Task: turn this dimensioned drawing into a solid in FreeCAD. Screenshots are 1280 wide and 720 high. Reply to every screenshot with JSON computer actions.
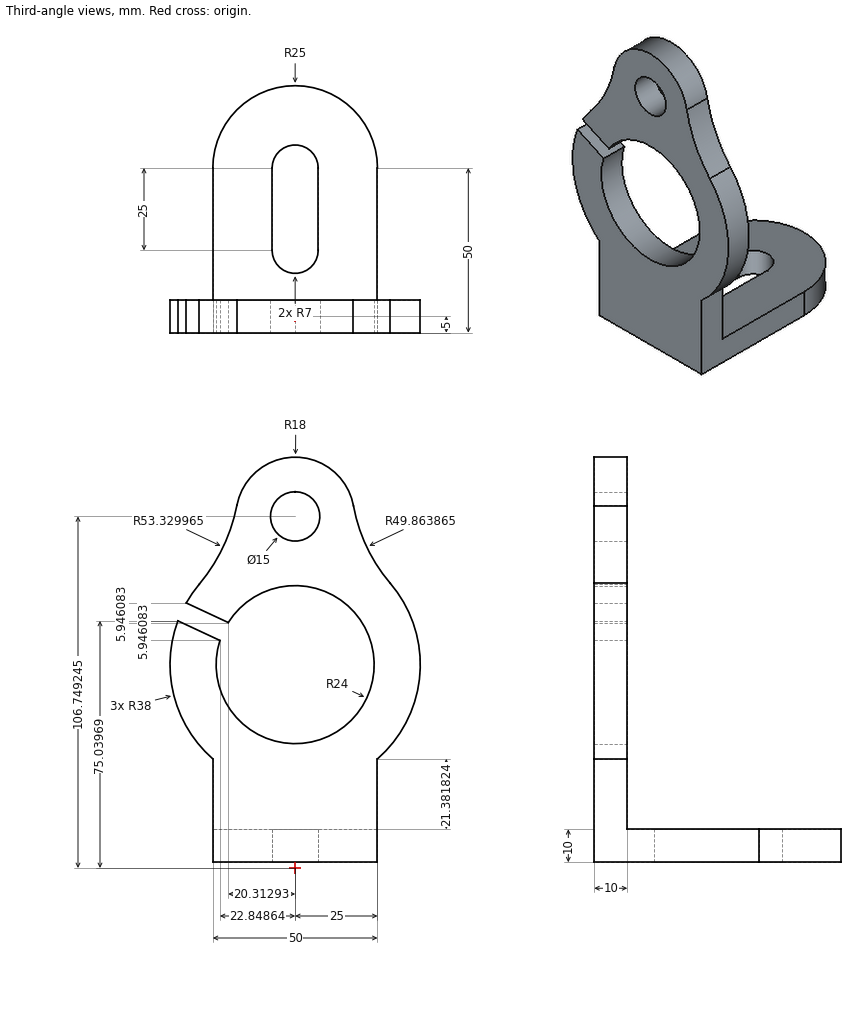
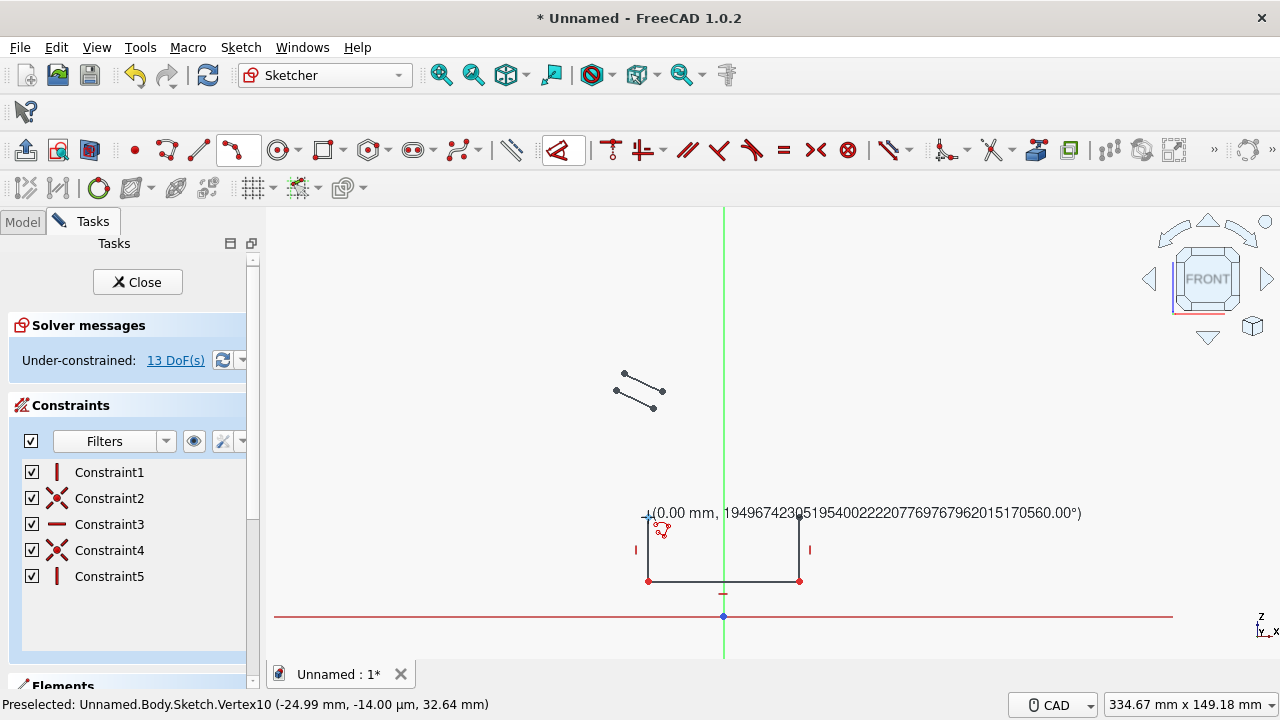
{"action": "left_click", "coordinate": [232, 150]}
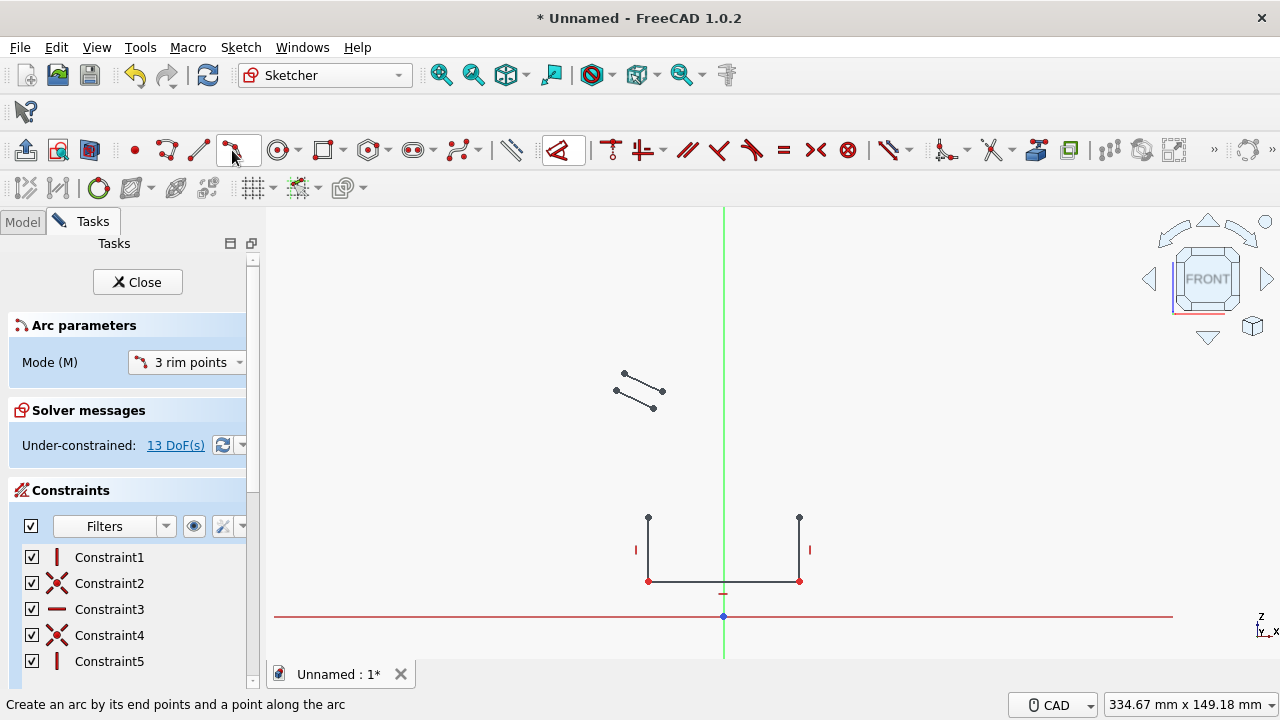
{"action": "left_click", "coordinate": [654, 409]}
{"action": "left_click", "coordinate": [662, 392]}
{"action": "left_click", "coordinate": [790, 461]}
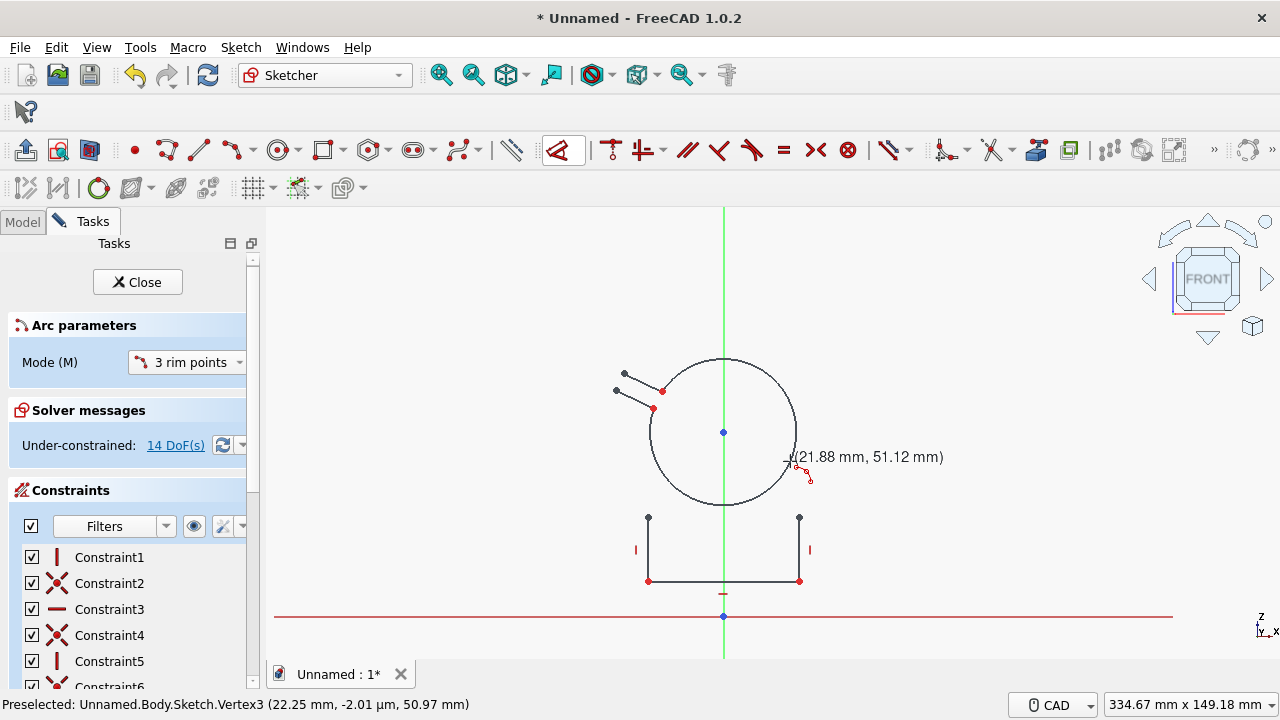
{"action": "left_click", "coordinate": [624, 374]}
{"action": "left_click", "coordinate": [635, 356]}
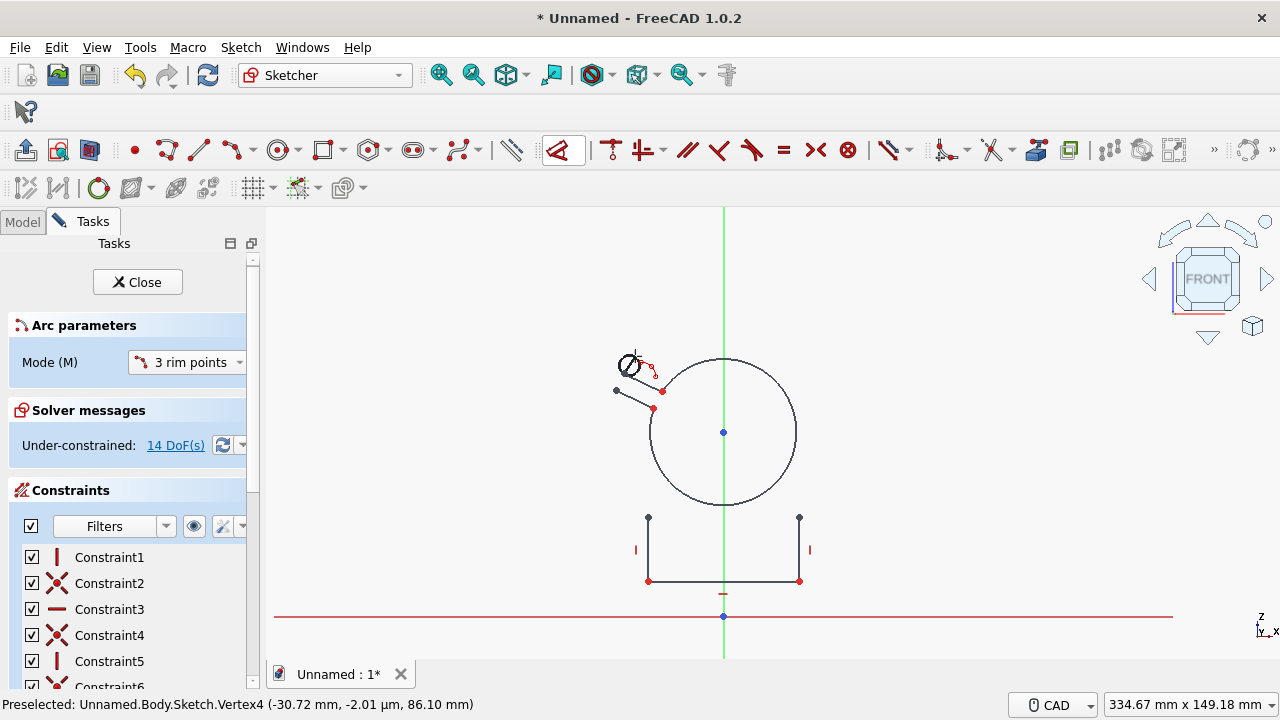
{"action": "scroll", "coordinate": [629, 364], "scroll_direction": "up", "scroll_amount": 18}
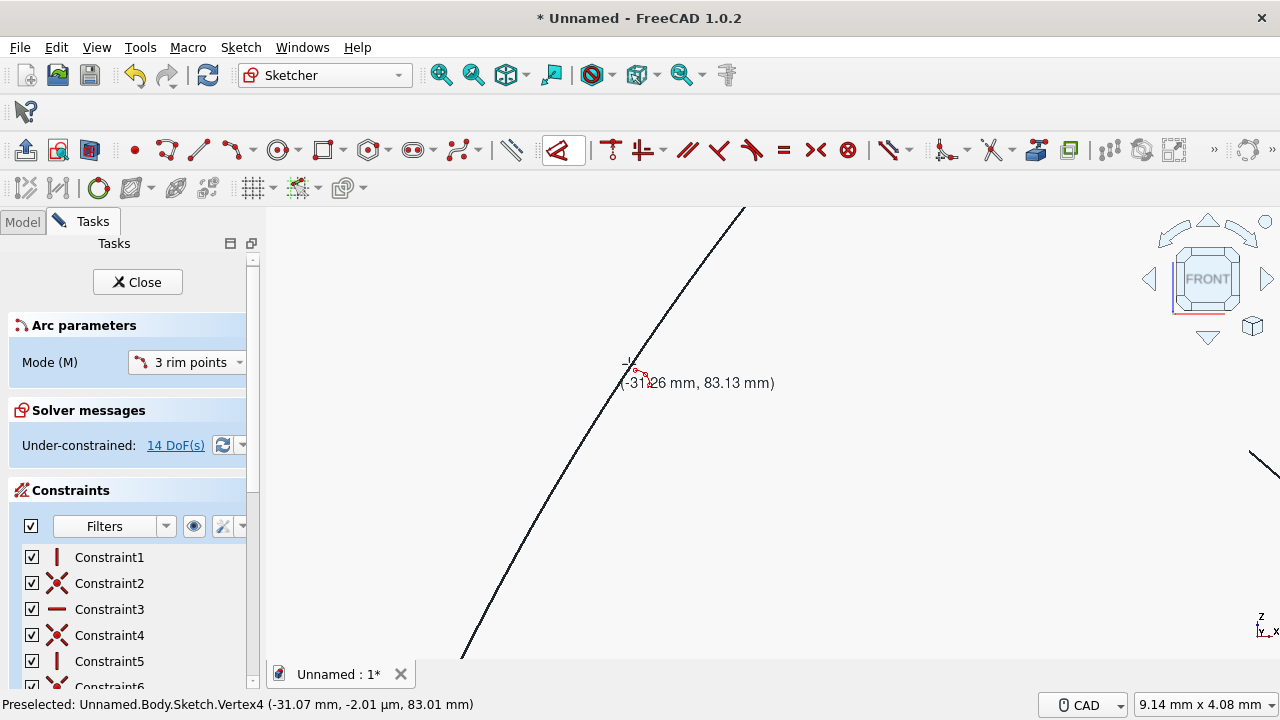
{"action": "left_click", "coordinate": [620, 358]}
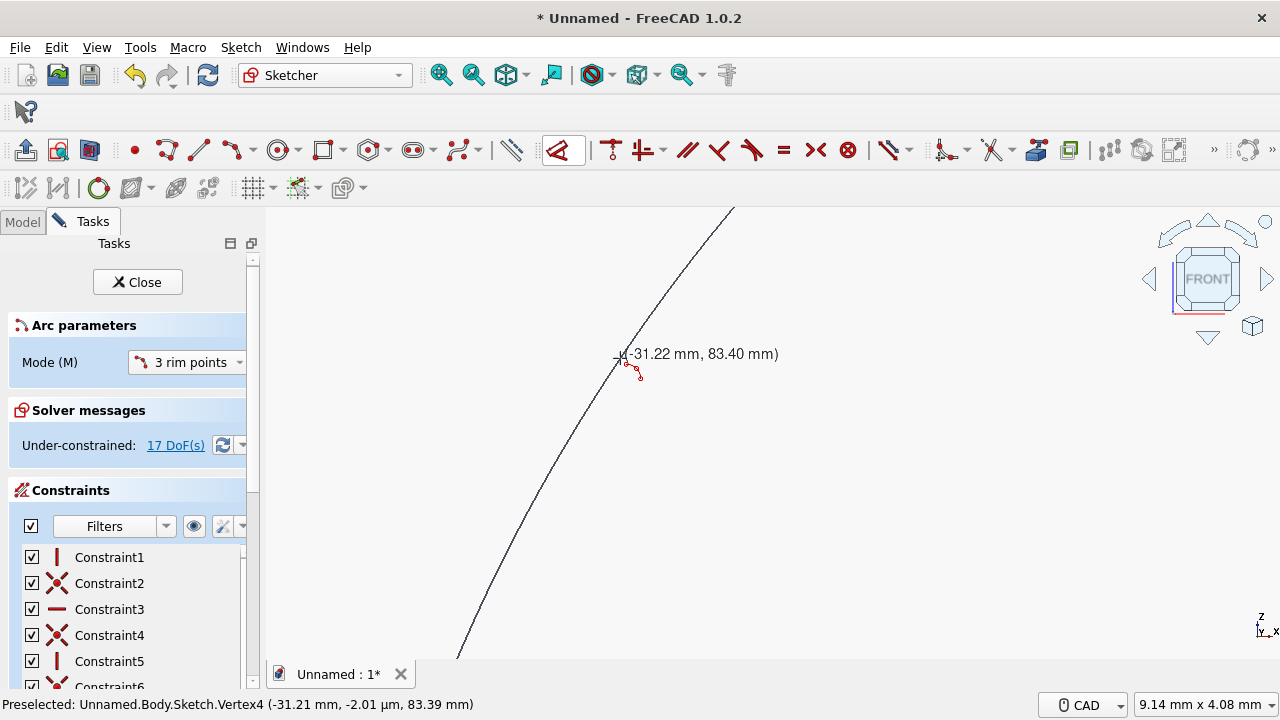
{"action": "scroll", "coordinate": [704, 433], "scroll_direction": "down", "scroll_amount": 15}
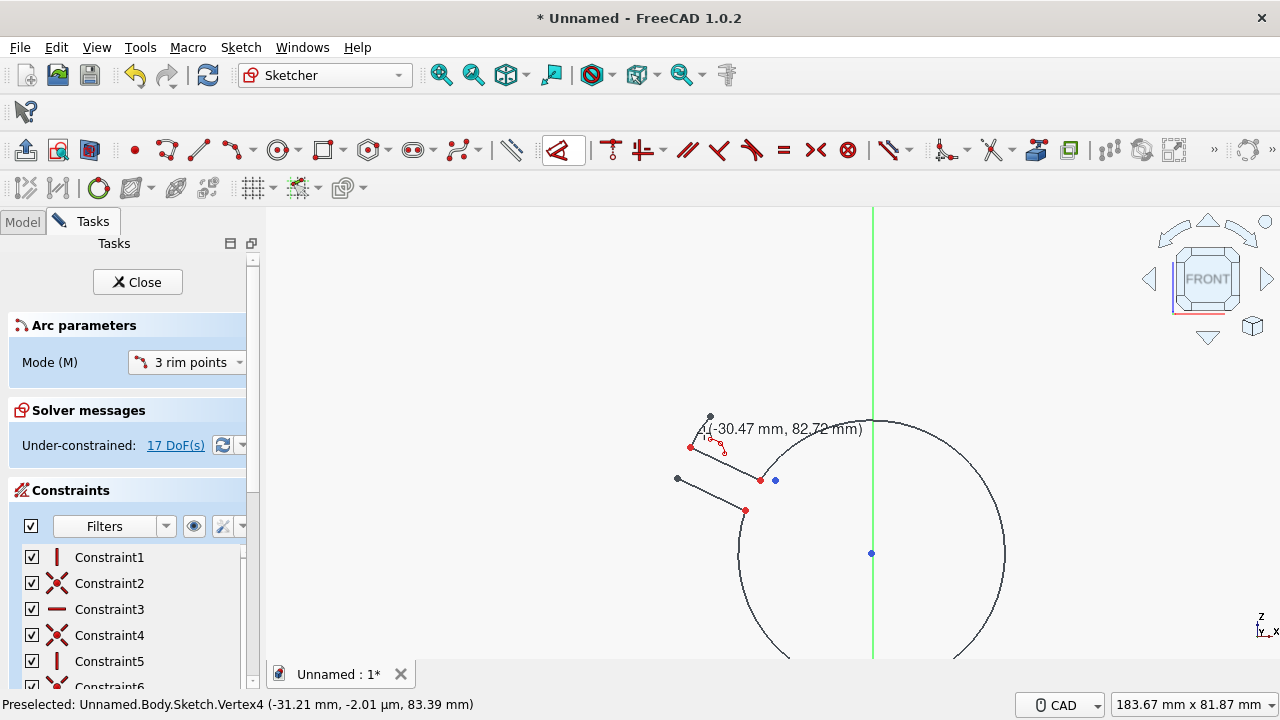
{"action": "scroll", "coordinate": [605, 367], "scroll_direction": "down", "scroll_amount": 5}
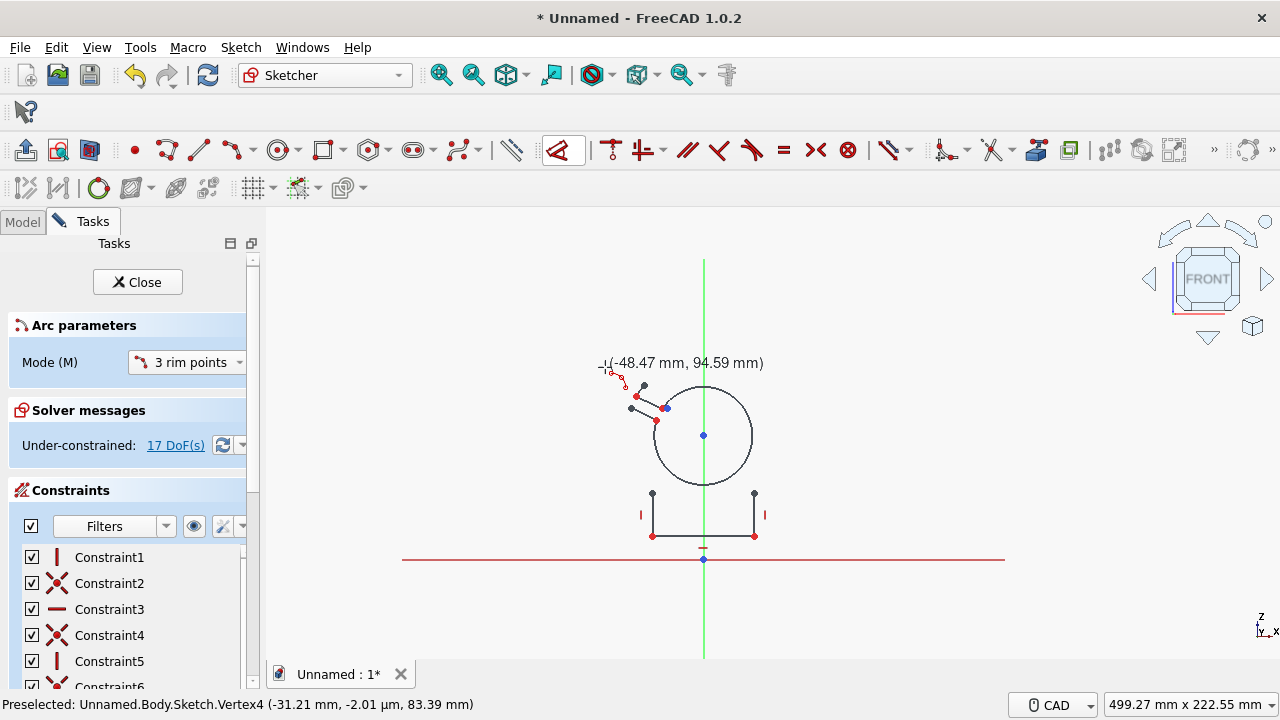
{"action": "left_click", "coordinate": [644, 385]}
{"action": "left_click", "coordinate": [668, 336]}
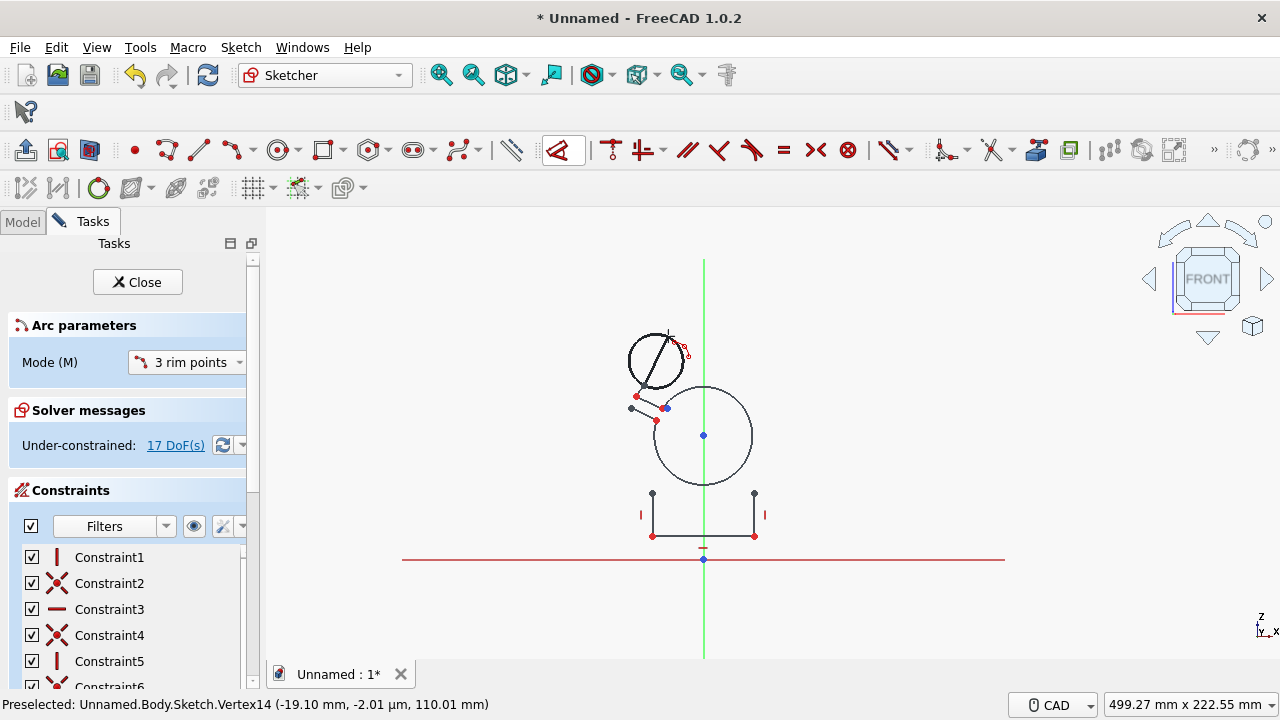
{"action": "scroll", "coordinate": [659, 362], "scroll_direction": "up", "scroll_amount": 8}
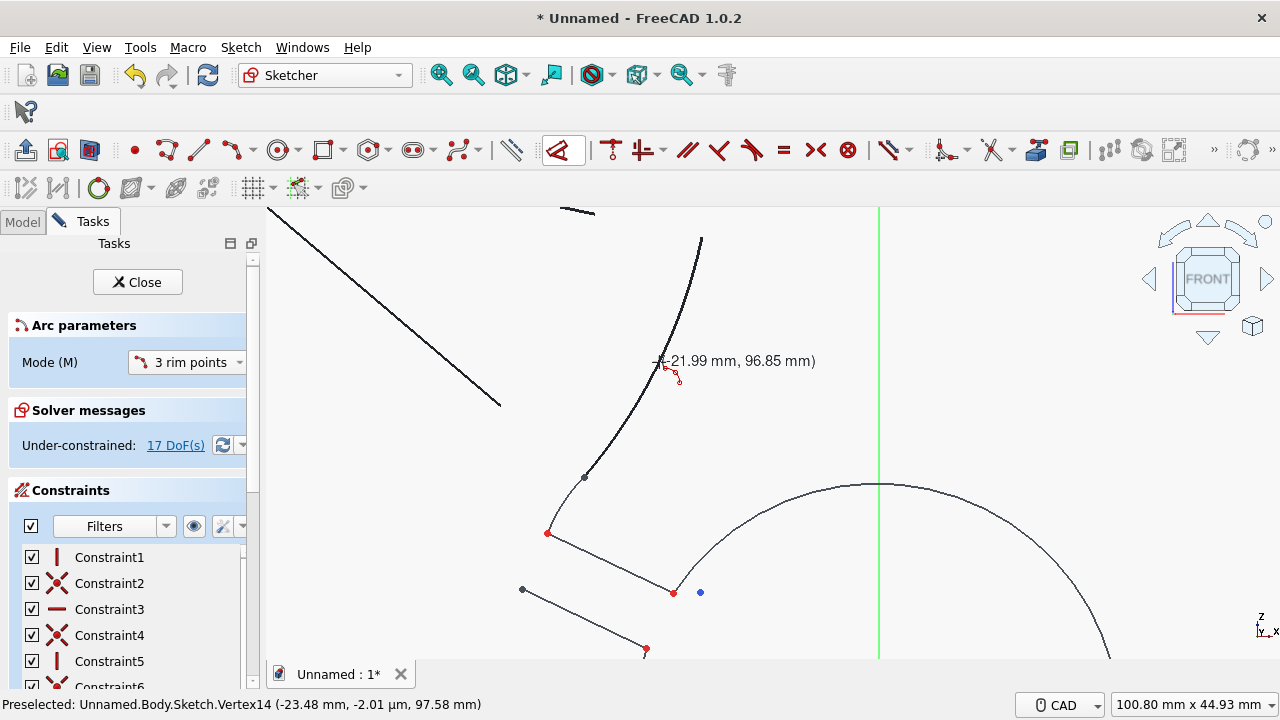
{"action": "left_click", "coordinate": [659, 360]}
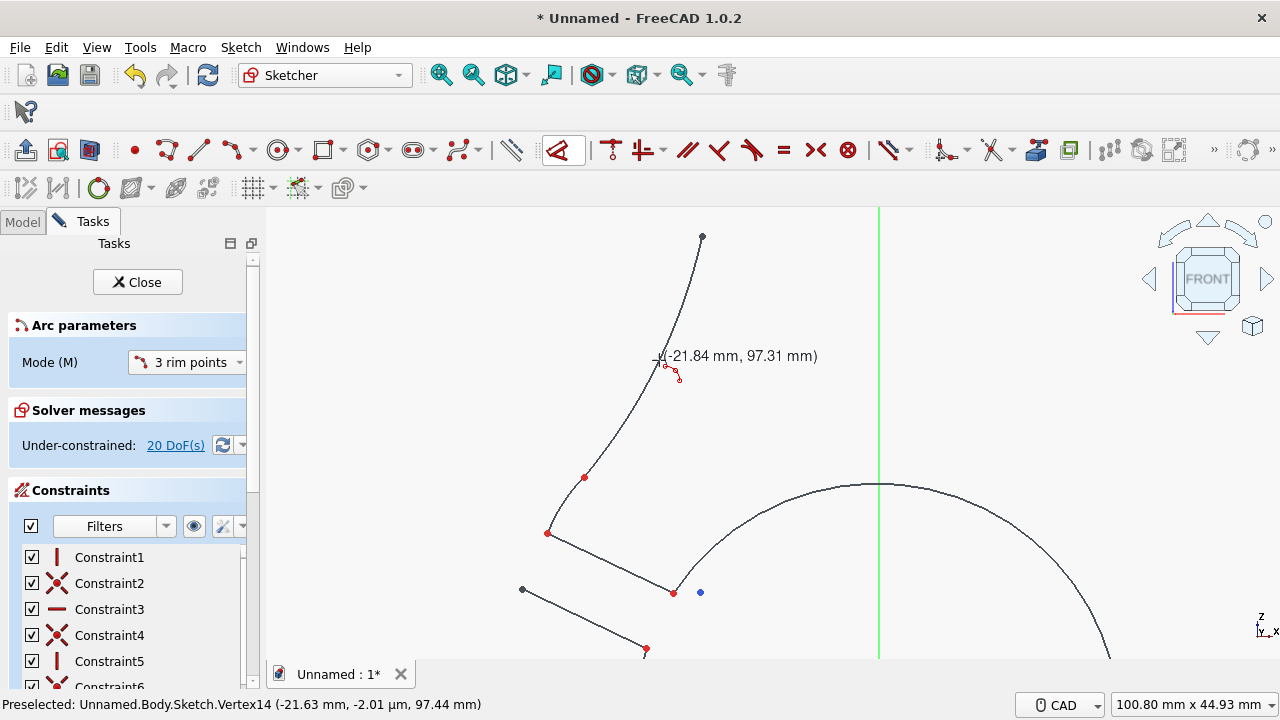
{"action": "scroll", "coordinate": [659, 362], "scroll_direction": "down", "scroll_amount": 8}